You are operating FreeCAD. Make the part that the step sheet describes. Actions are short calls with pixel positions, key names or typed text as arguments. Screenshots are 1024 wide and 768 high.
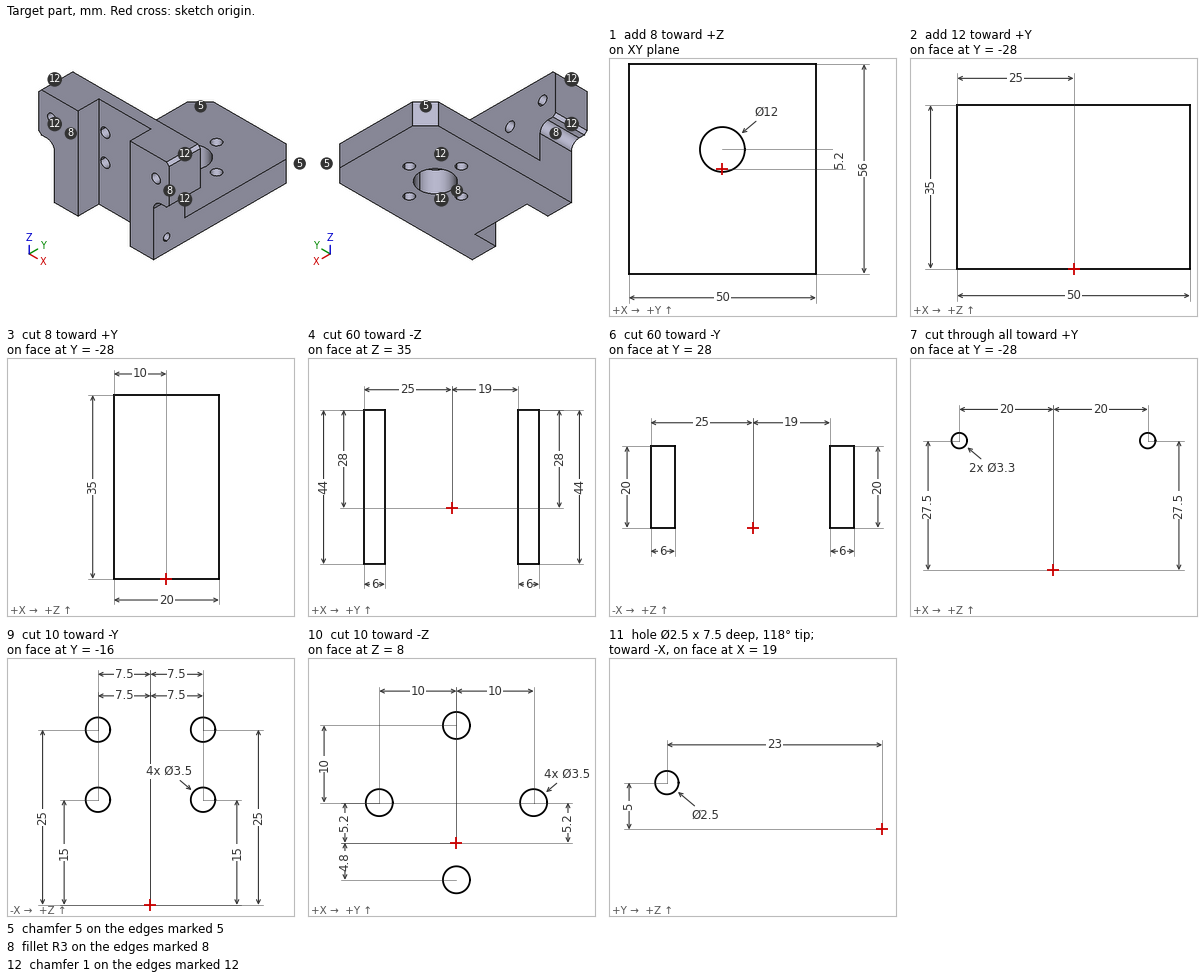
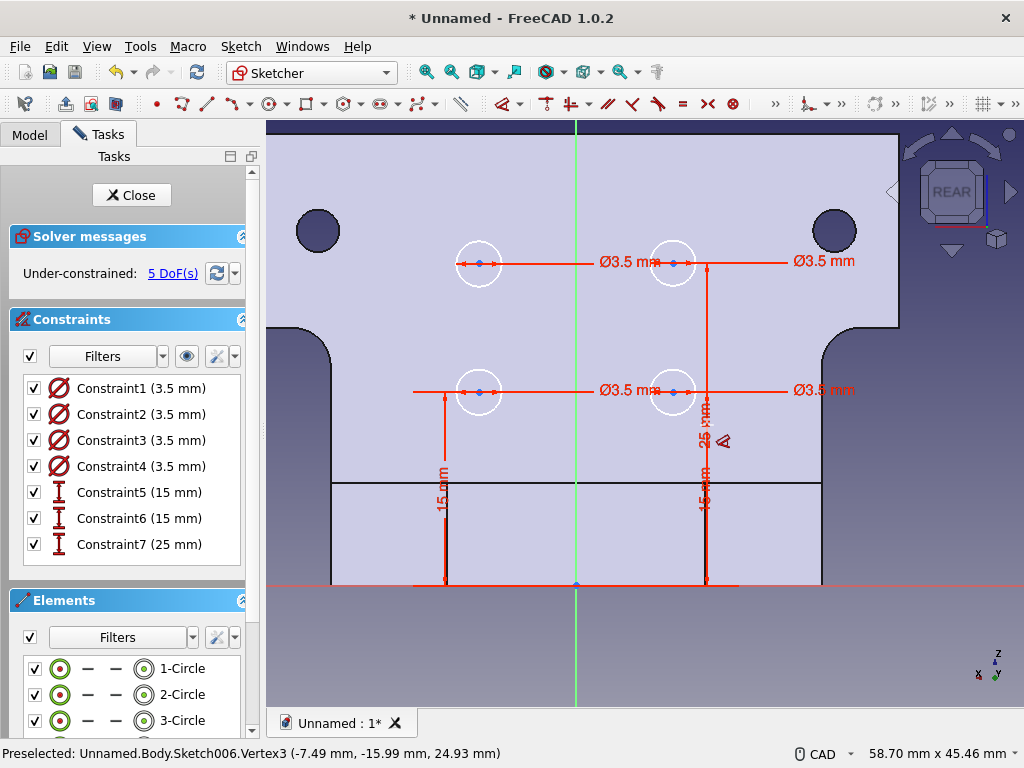
click(479, 264)
click(445, 425)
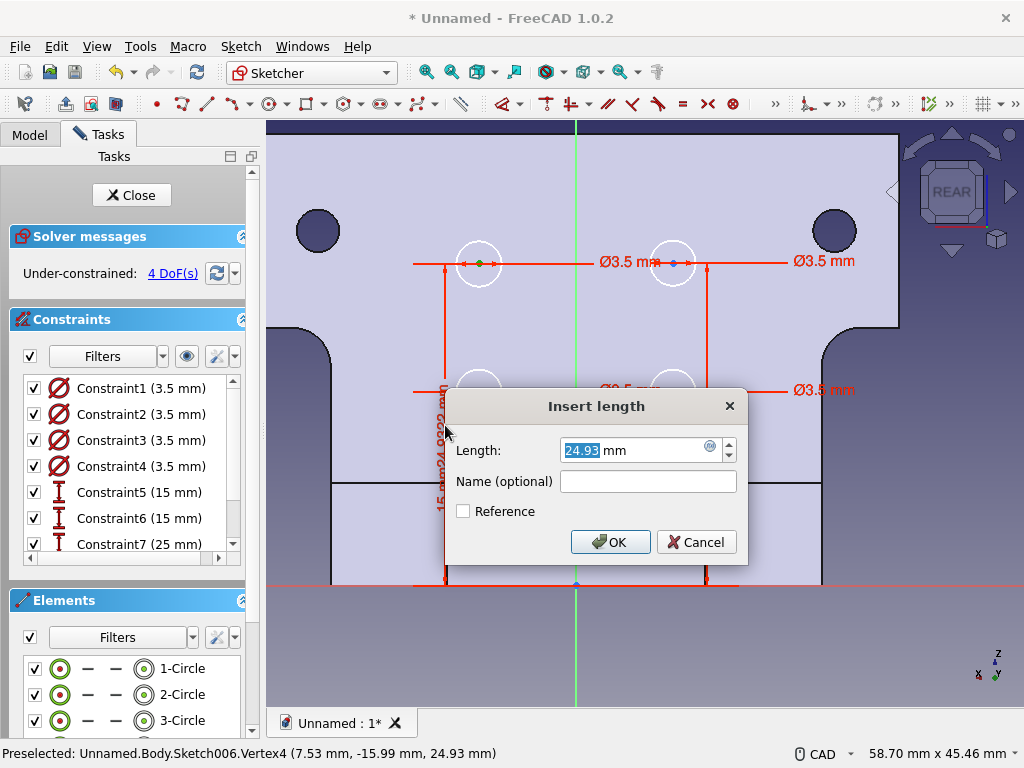
text(25)
key(Return)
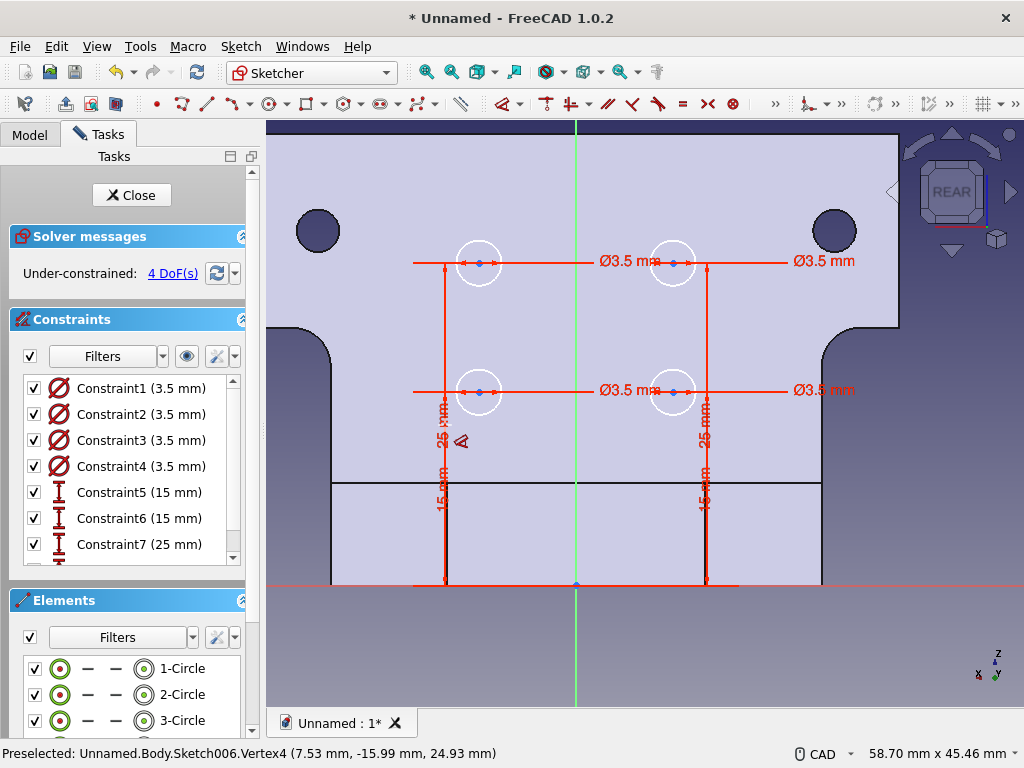
click(673, 392)
click(625, 620)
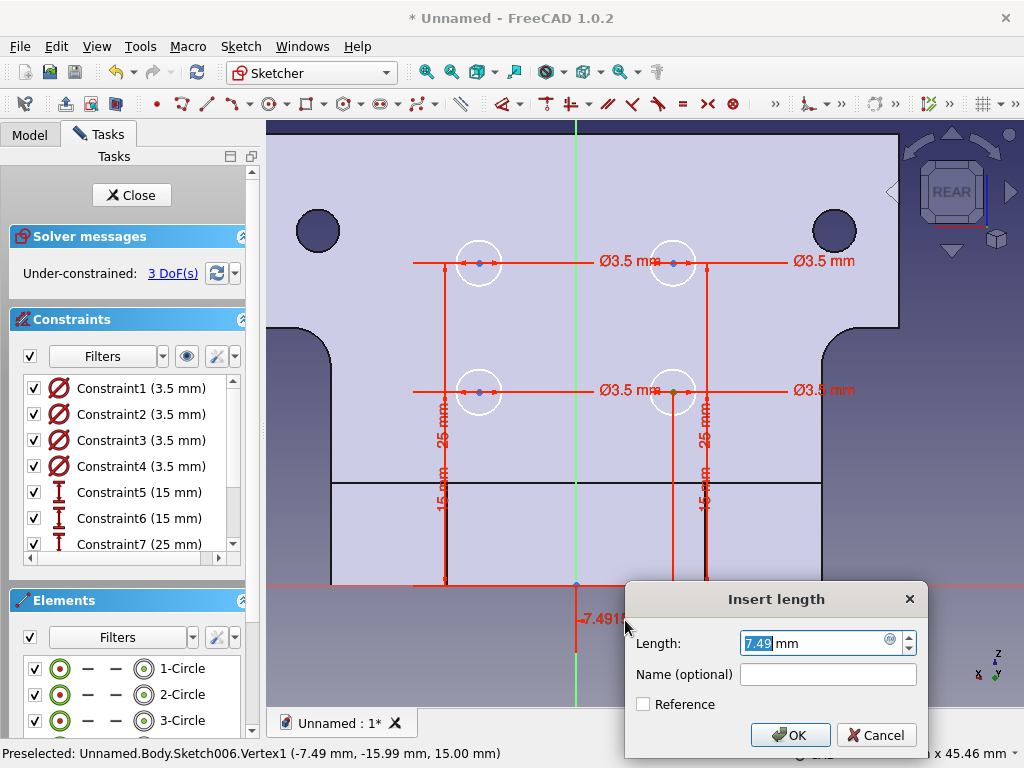
text(7.5)
key(Return)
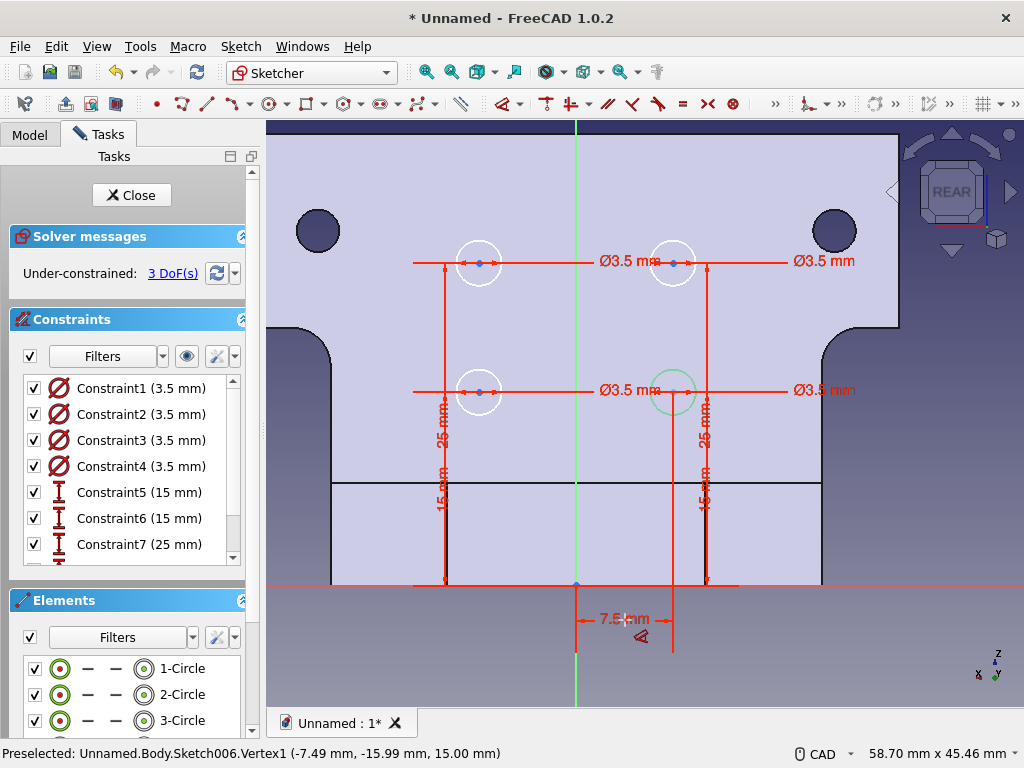
click(479, 392)
click(528, 620)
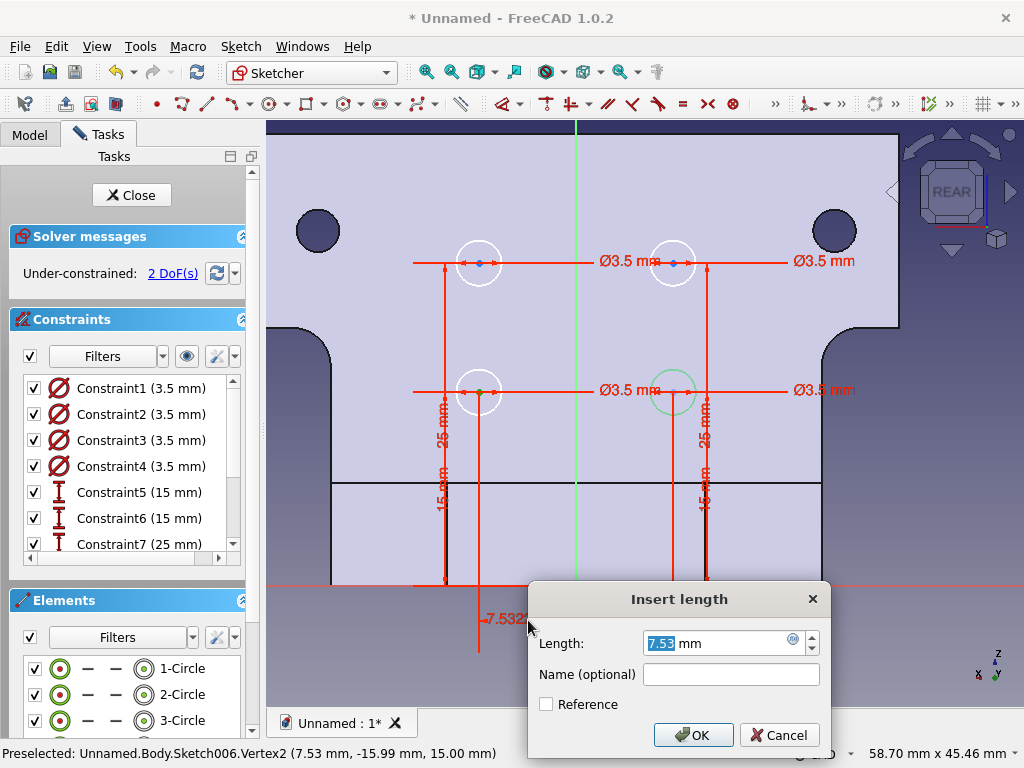
text(7.5)
key(Return)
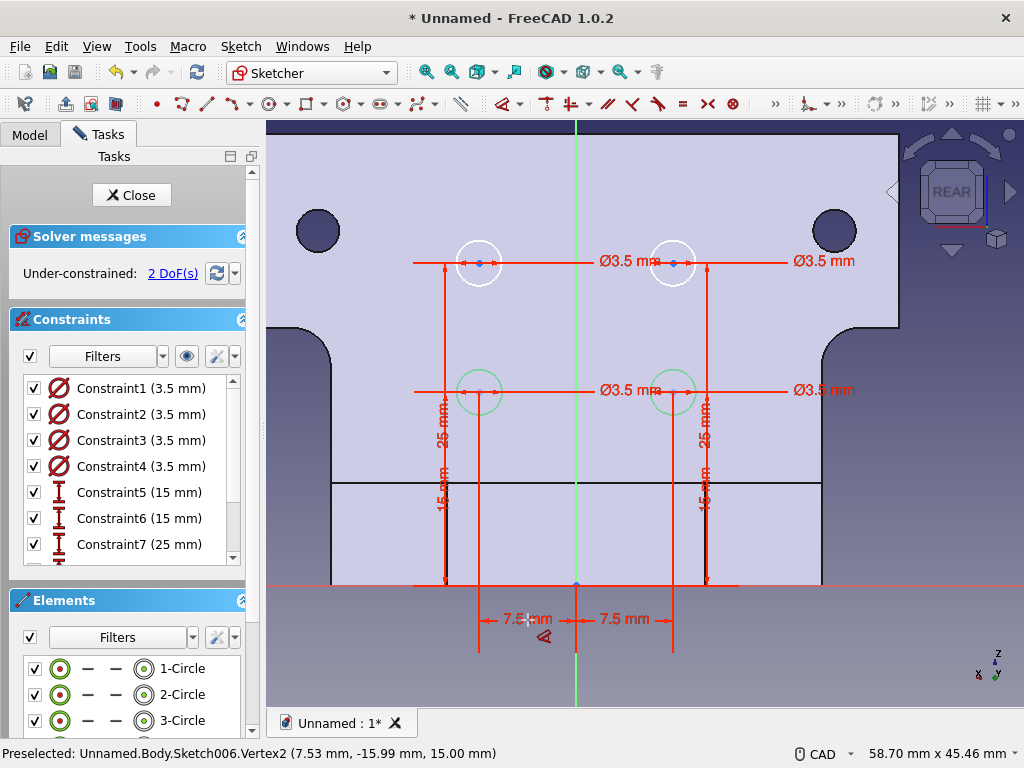
click(673, 263)
click(625, 229)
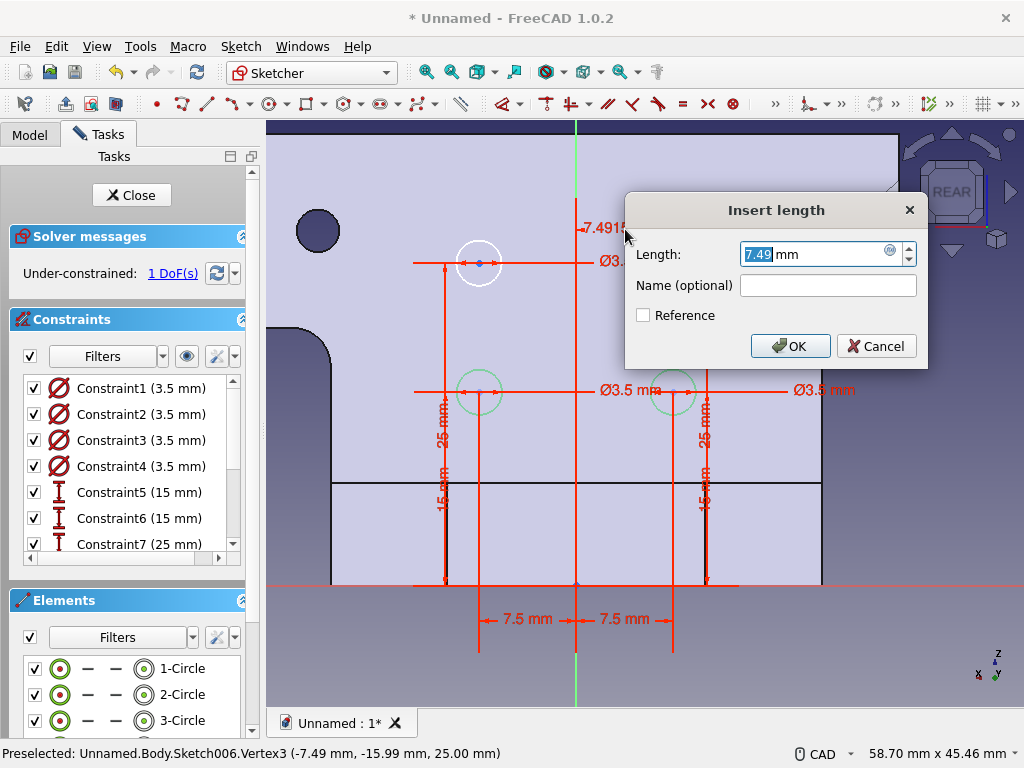
text(7.5)
key(Return)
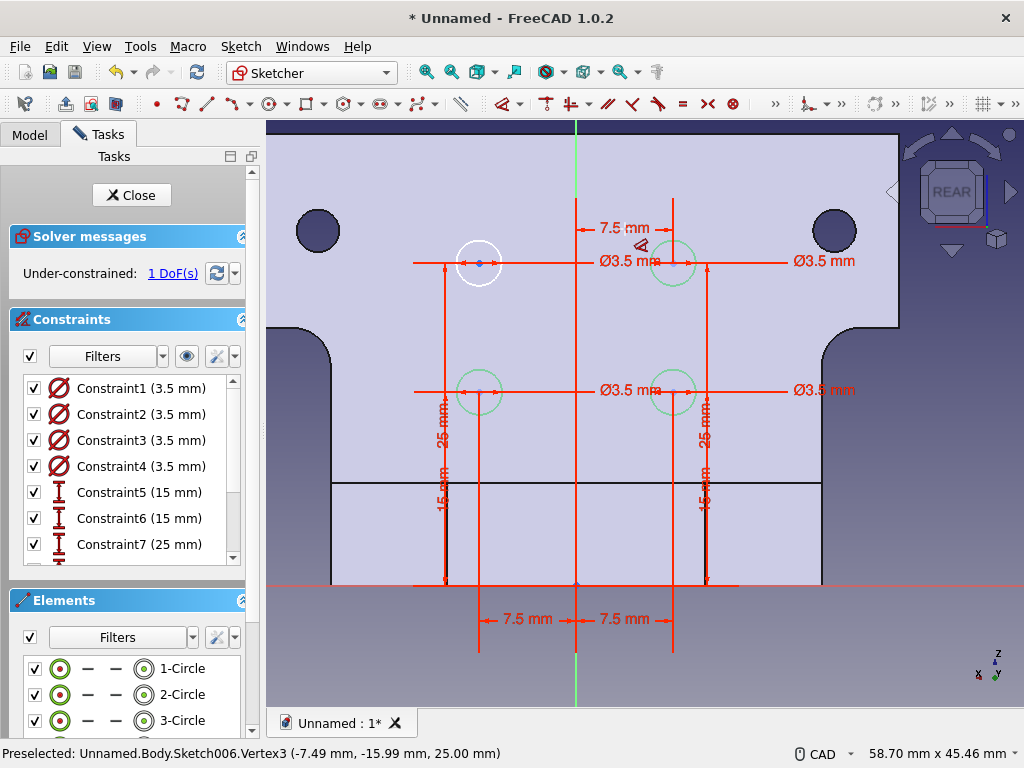
click(479, 263)
click(528, 229)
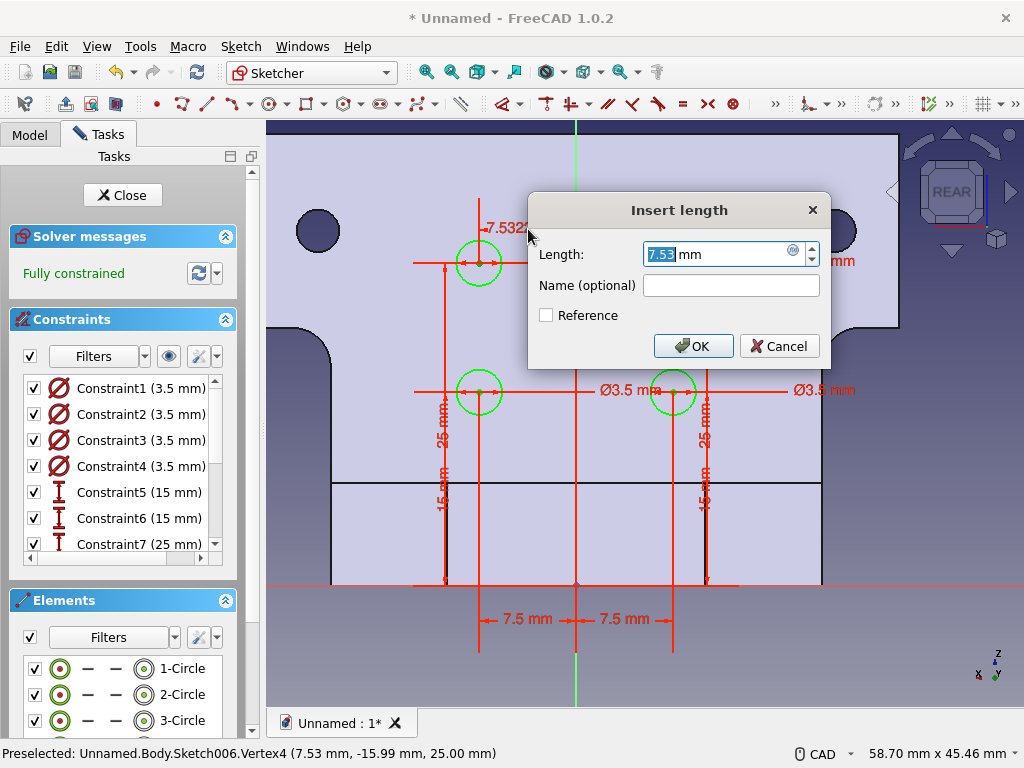
text(7.5)
key(Return)
key(Escape)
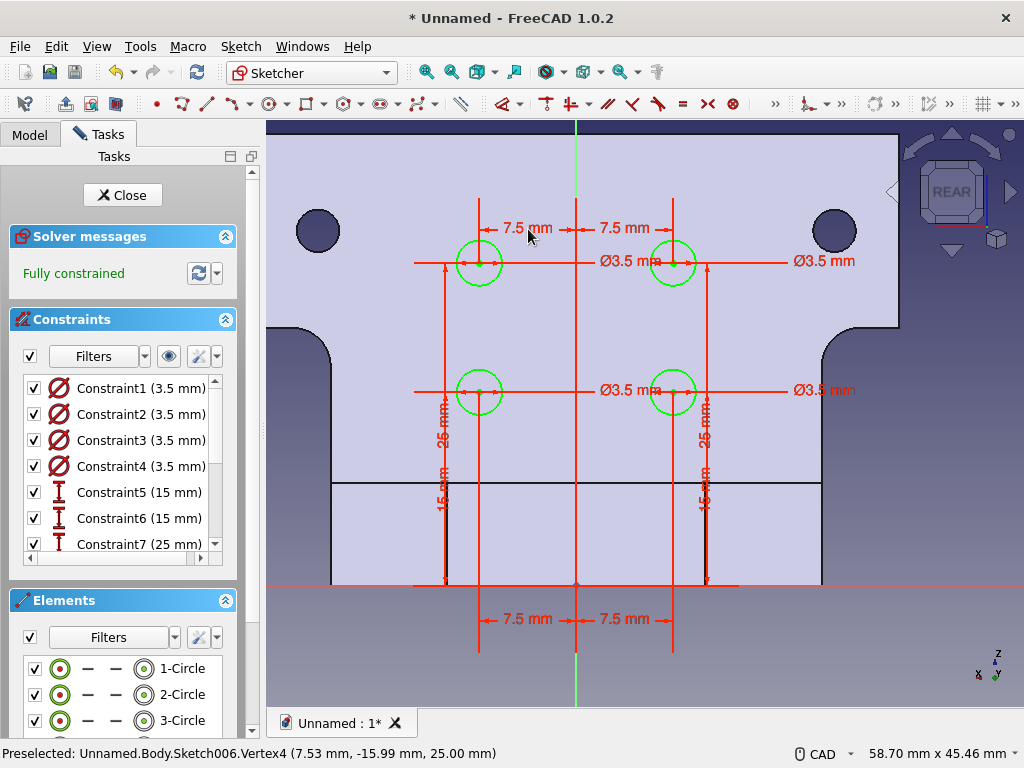
click(123, 195)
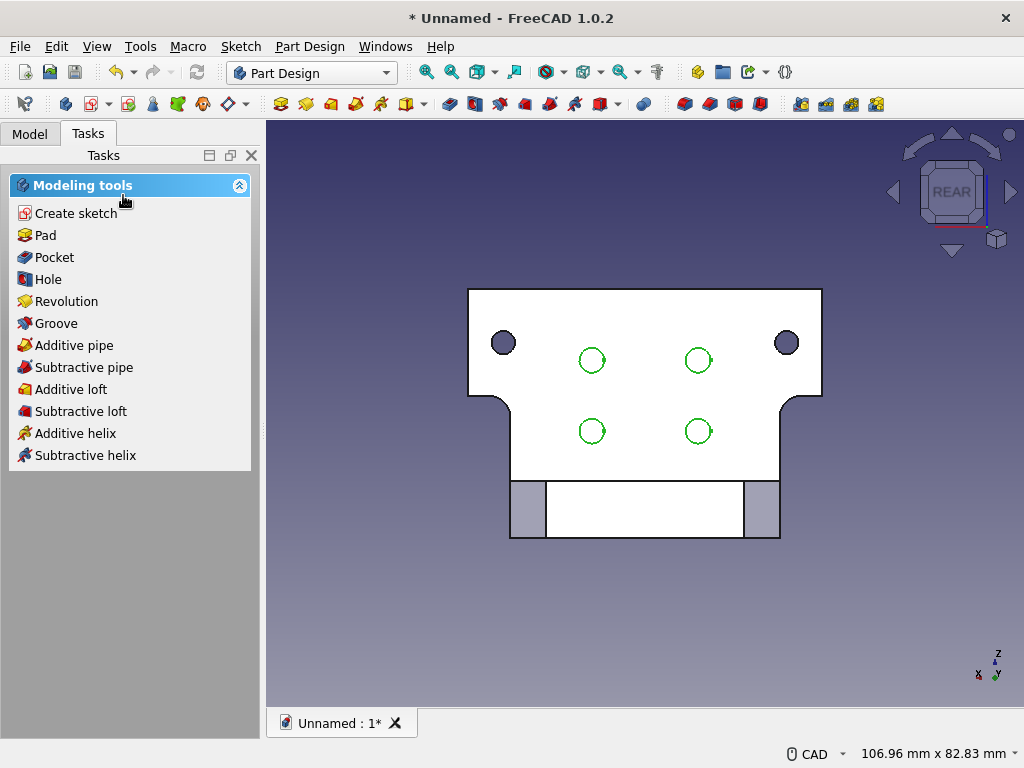
click(450, 104)